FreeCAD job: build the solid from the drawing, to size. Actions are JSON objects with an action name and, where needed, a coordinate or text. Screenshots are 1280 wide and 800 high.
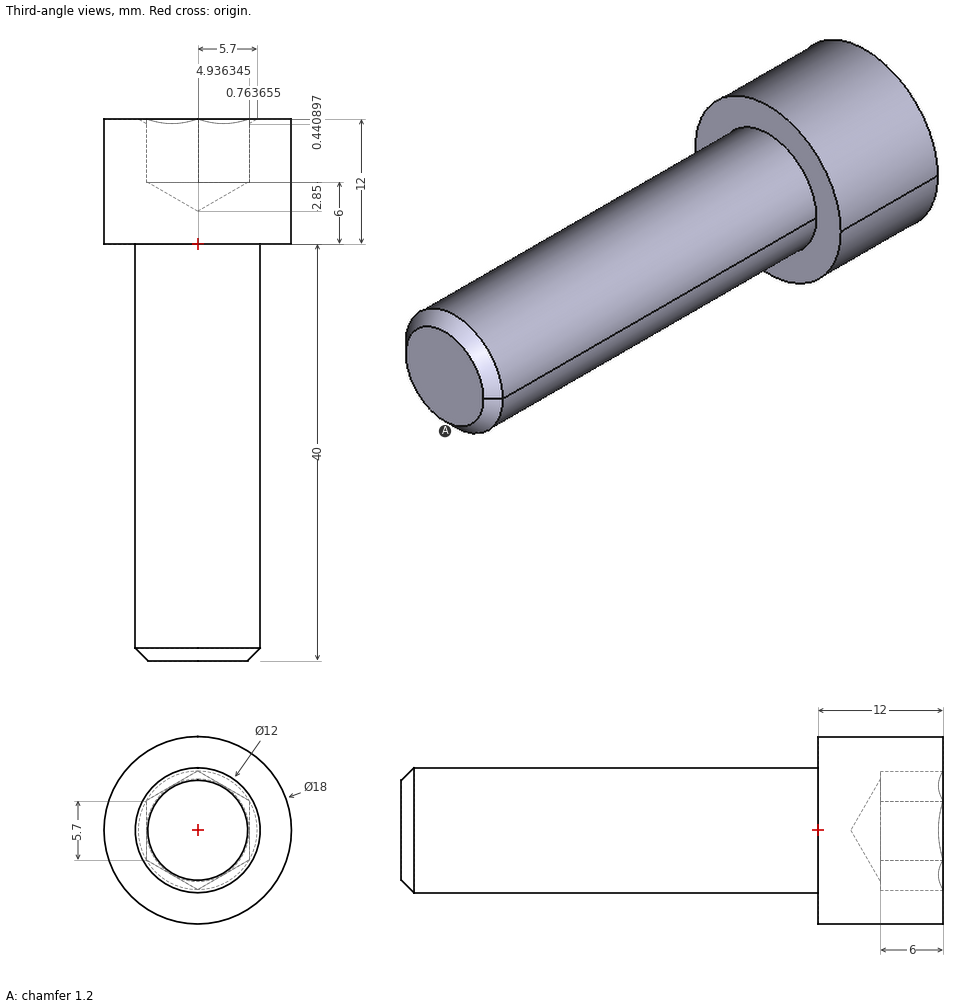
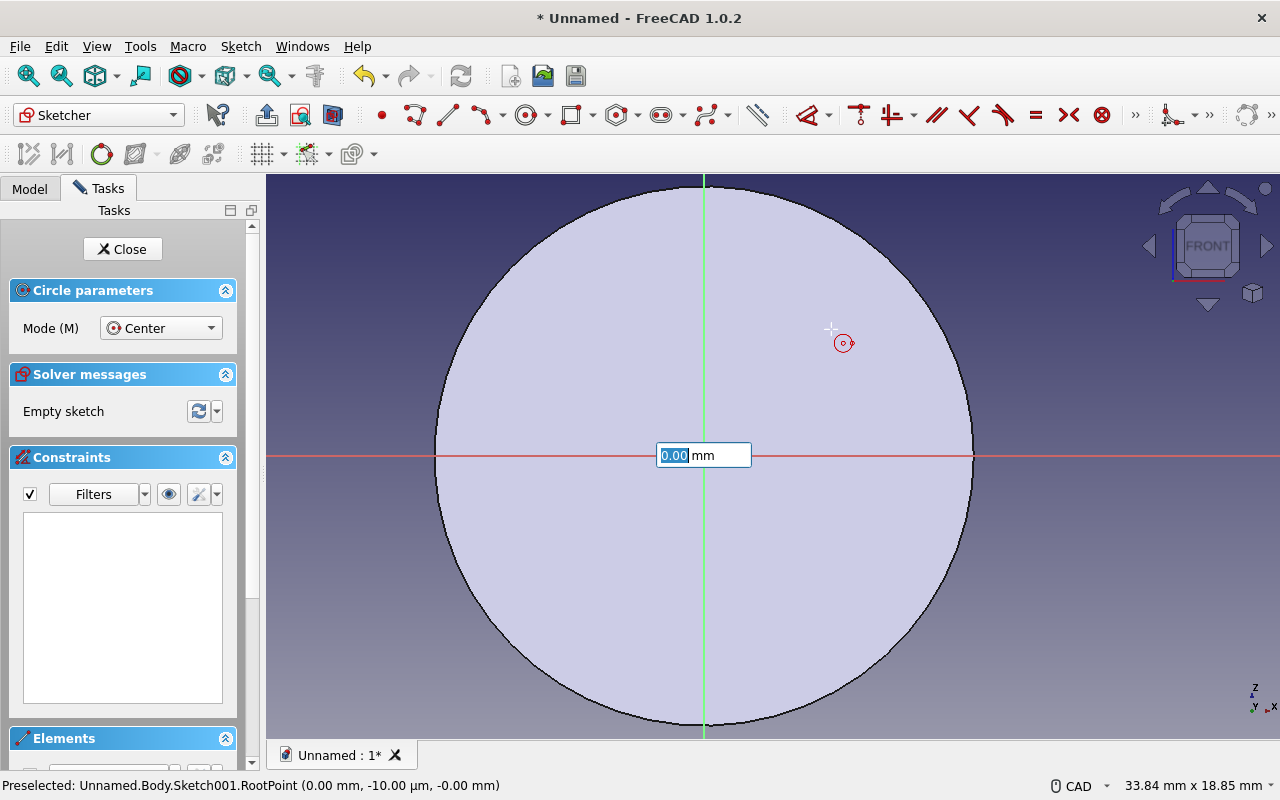
{"action": "type", "text": "12"}
{"action": "key", "text": "Return"}
{"action": "key", "text": "Escape"}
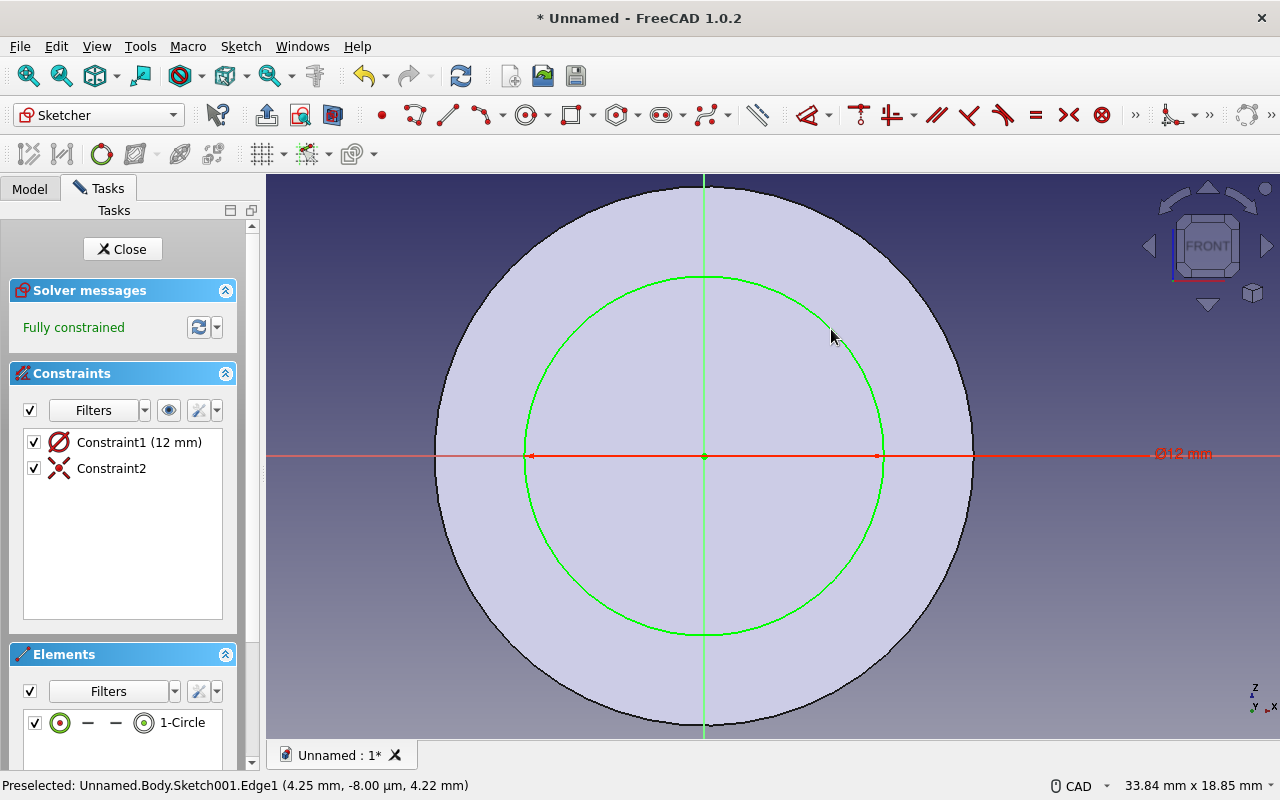
{"action": "left_click", "coordinate": [123, 249]}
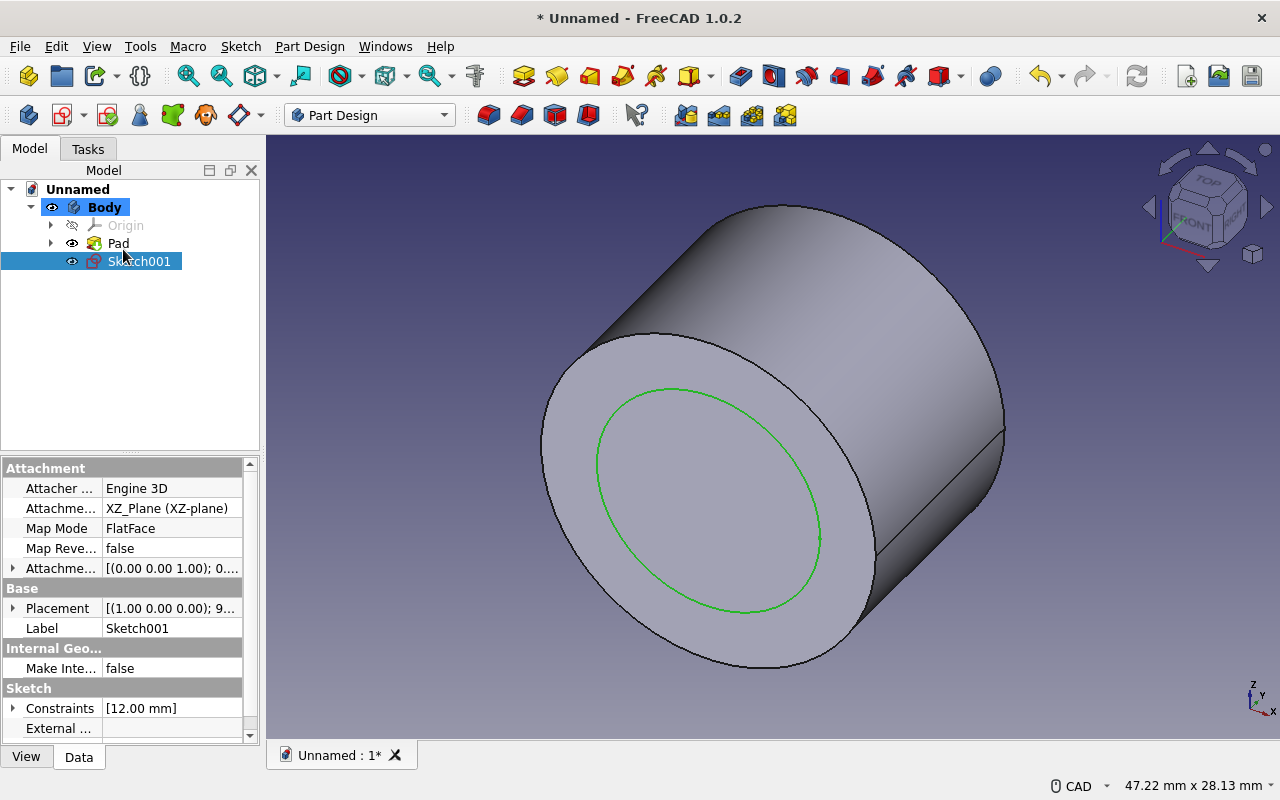
{"action": "left_click", "coordinate": [524, 76]}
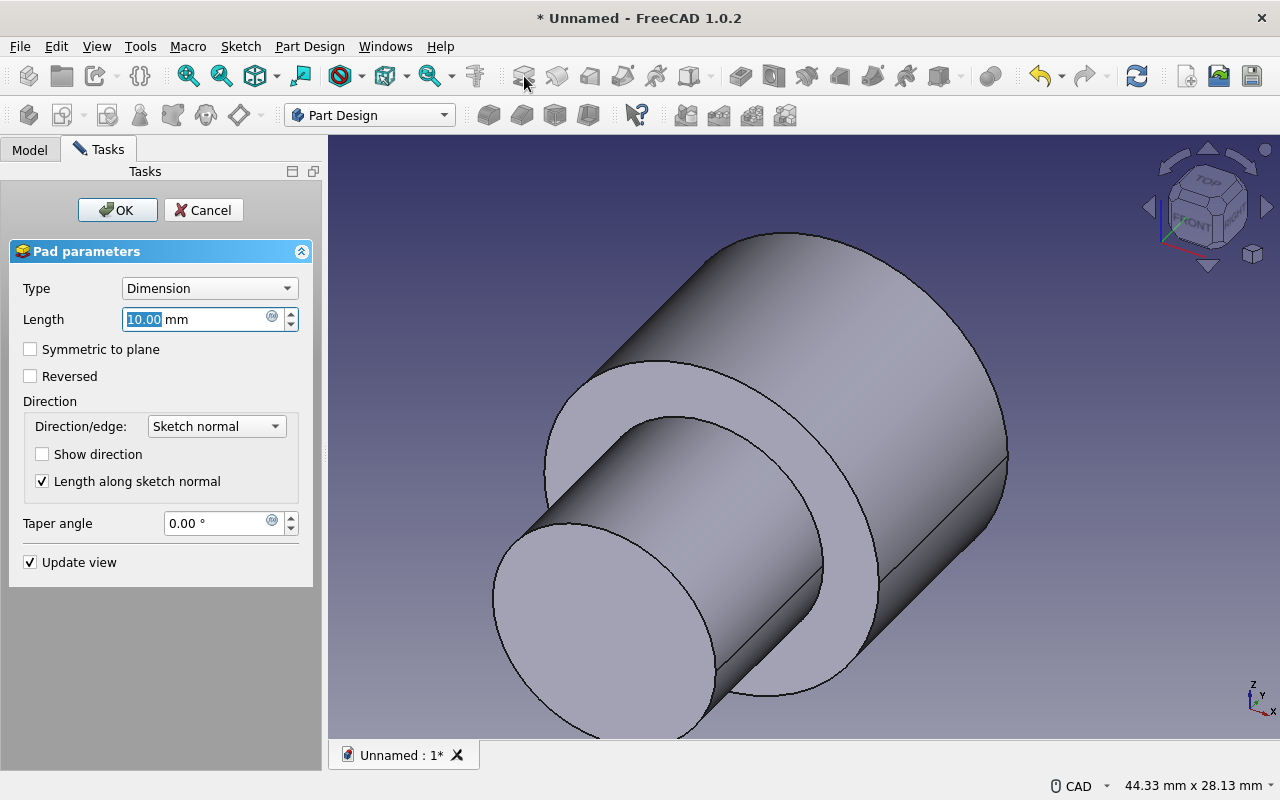
{"action": "type", "text": "40"}
{"action": "key", "text": "Tab"}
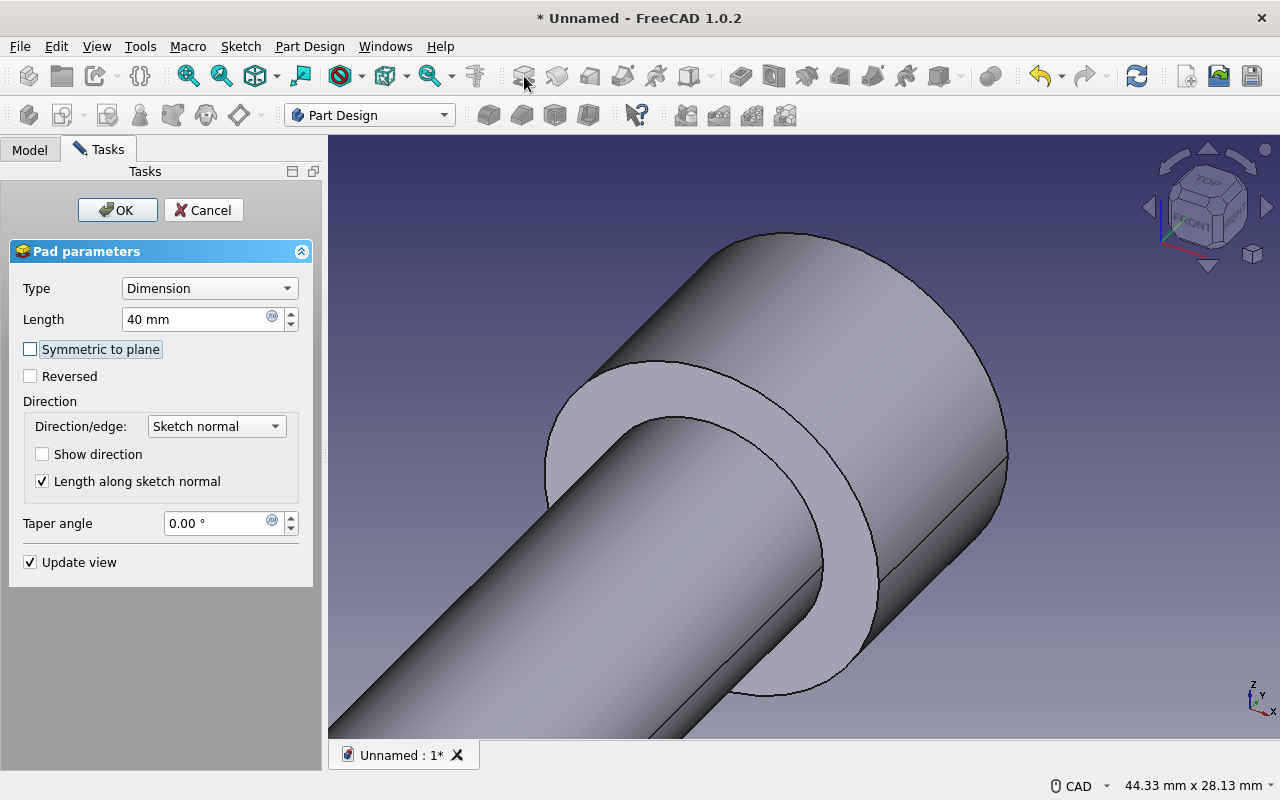
{"action": "left_click", "coordinate": [118, 210]}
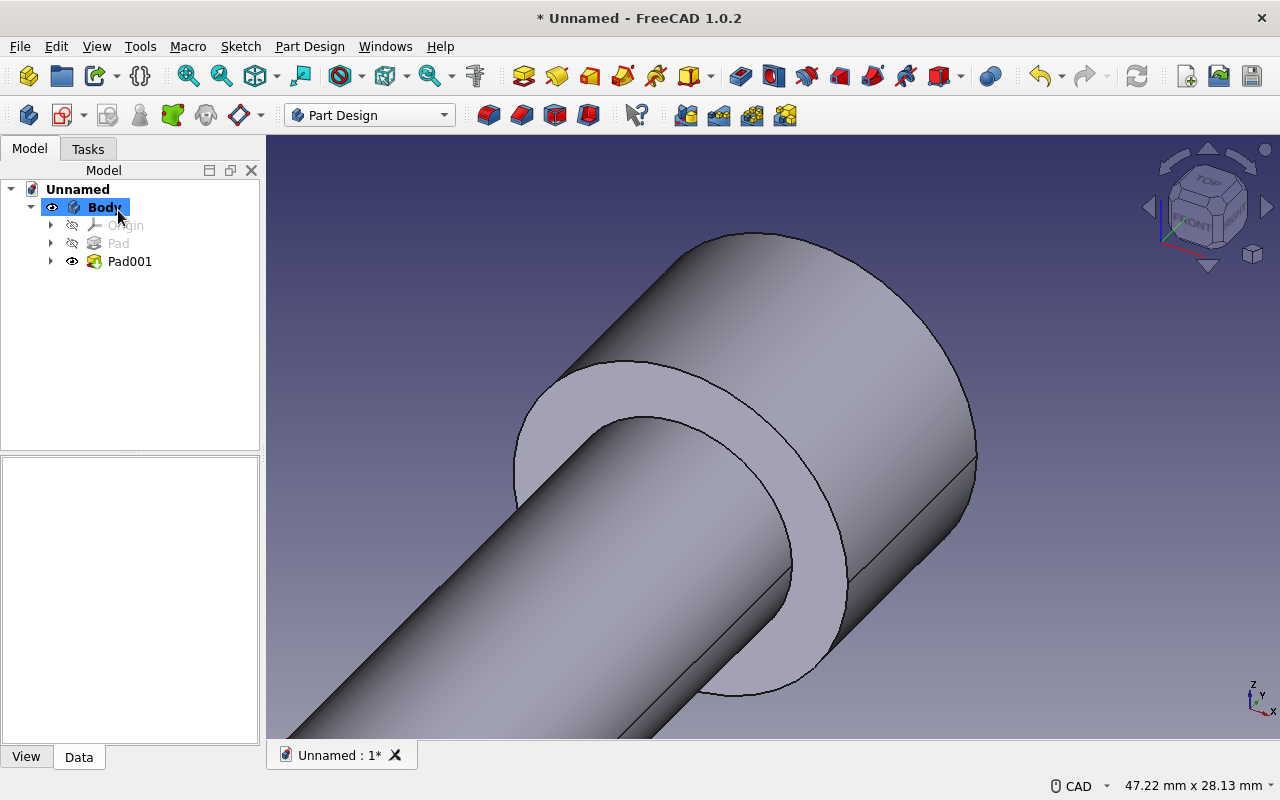
{"action": "left_click", "coordinate": [189, 76]}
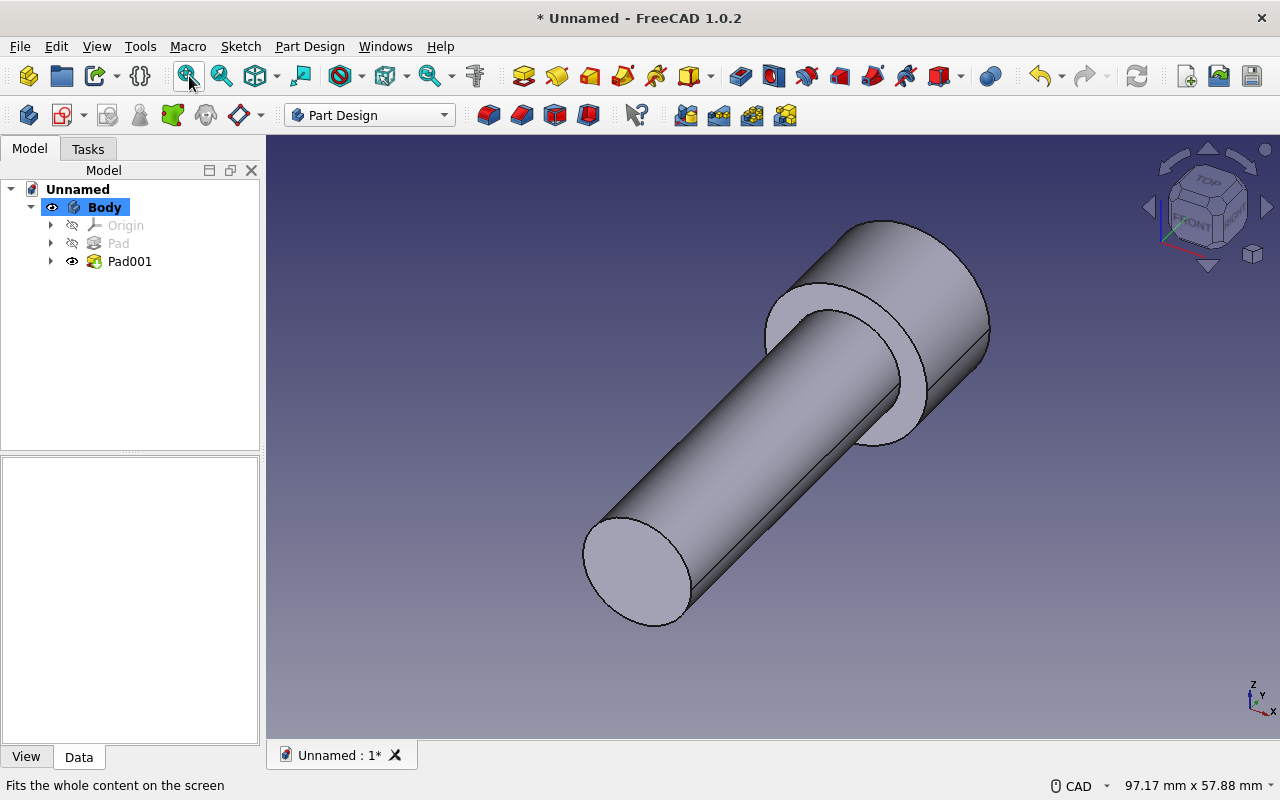
{"action": "key", "text": "4"}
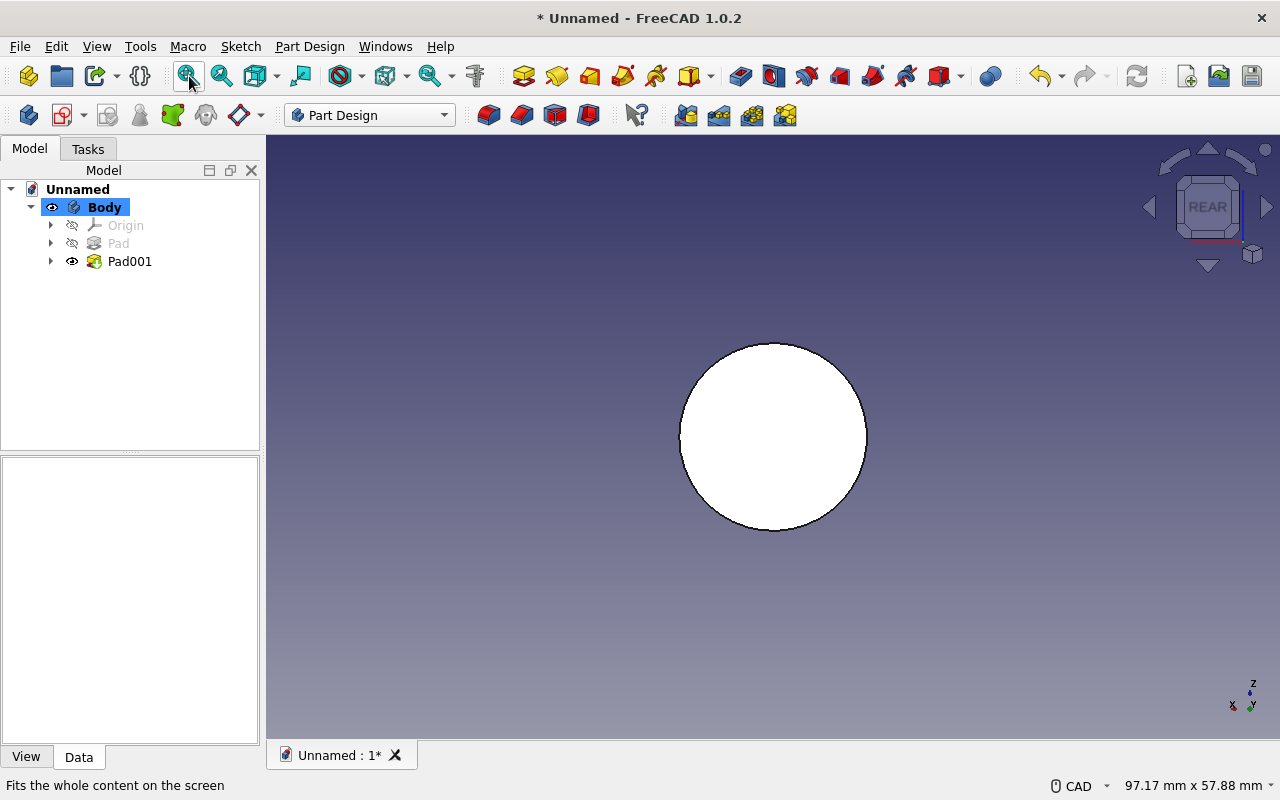
{"action": "left_click", "coordinate": [189, 76]}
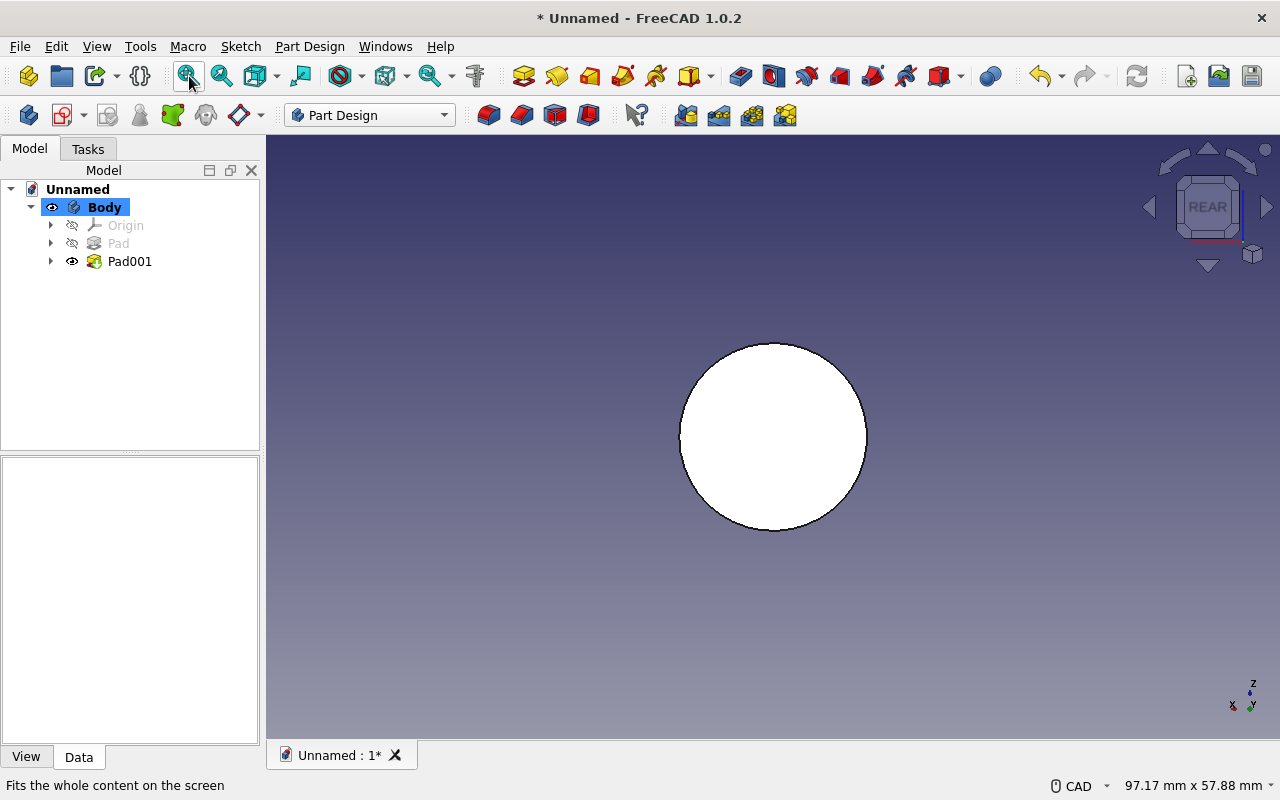
{"action": "left_click", "coordinate": [773, 436]}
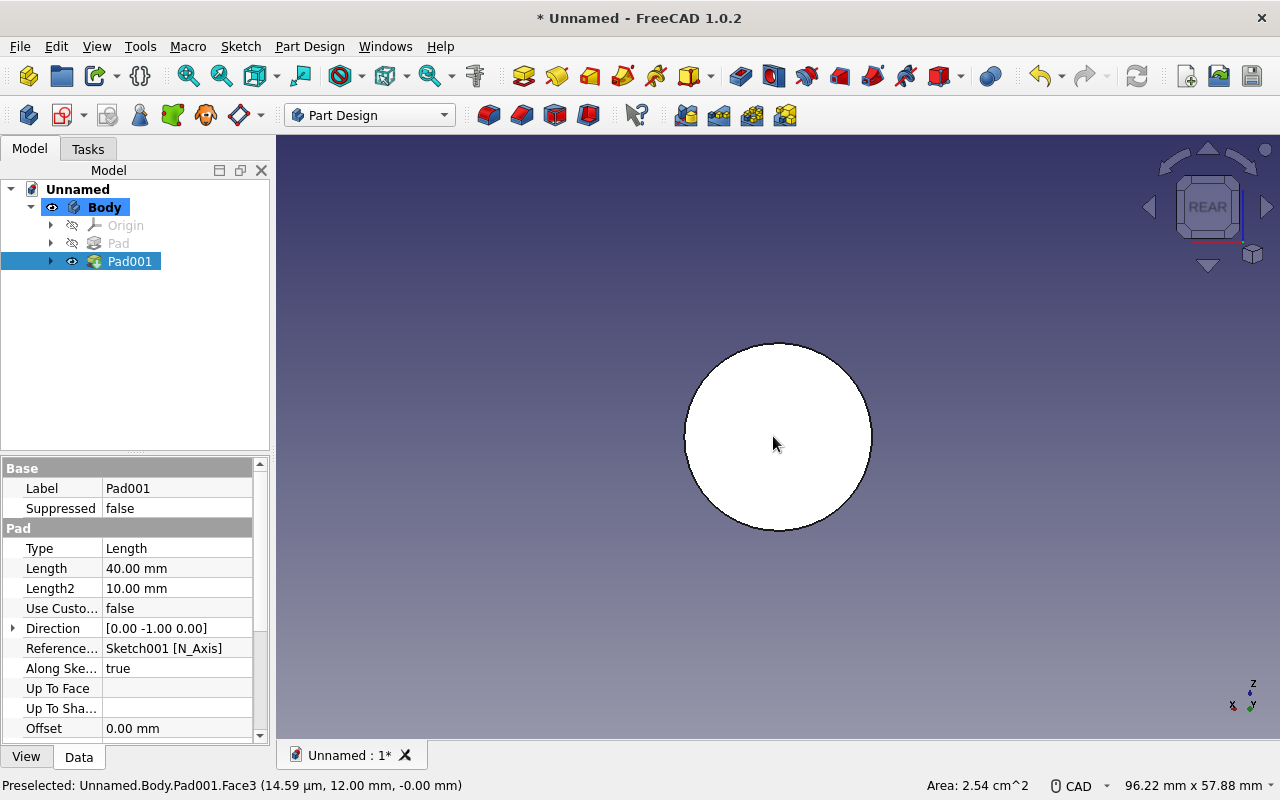
{"action": "left_click", "coordinate": [62, 116]}